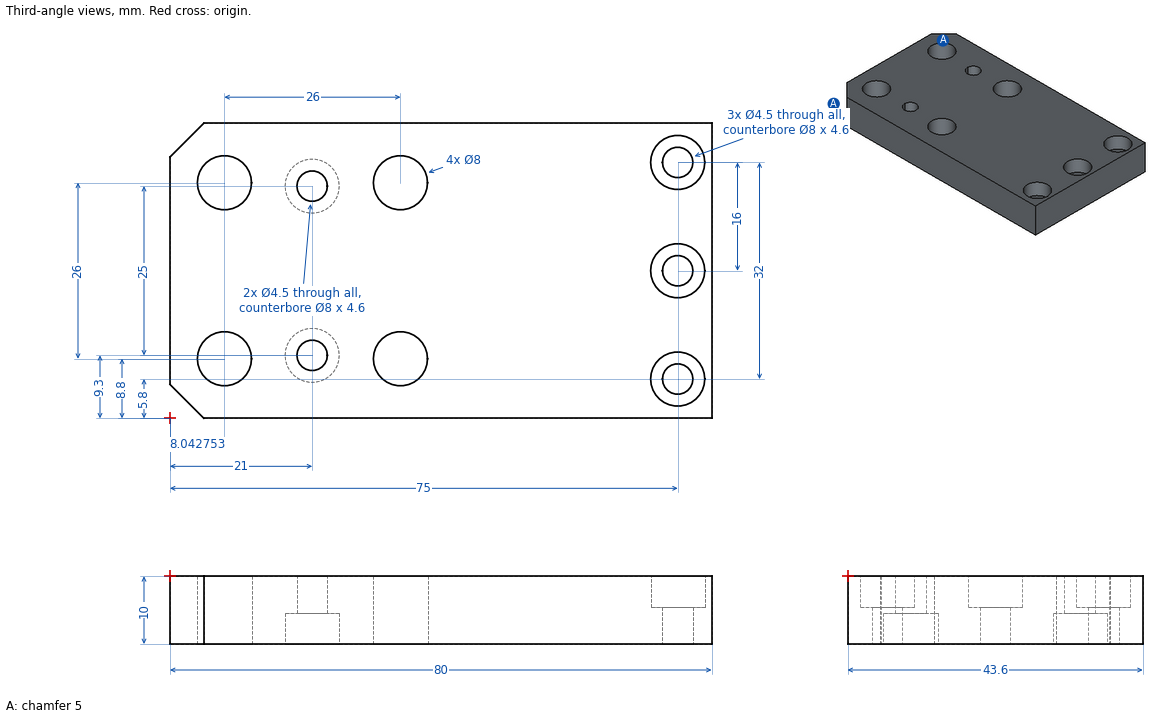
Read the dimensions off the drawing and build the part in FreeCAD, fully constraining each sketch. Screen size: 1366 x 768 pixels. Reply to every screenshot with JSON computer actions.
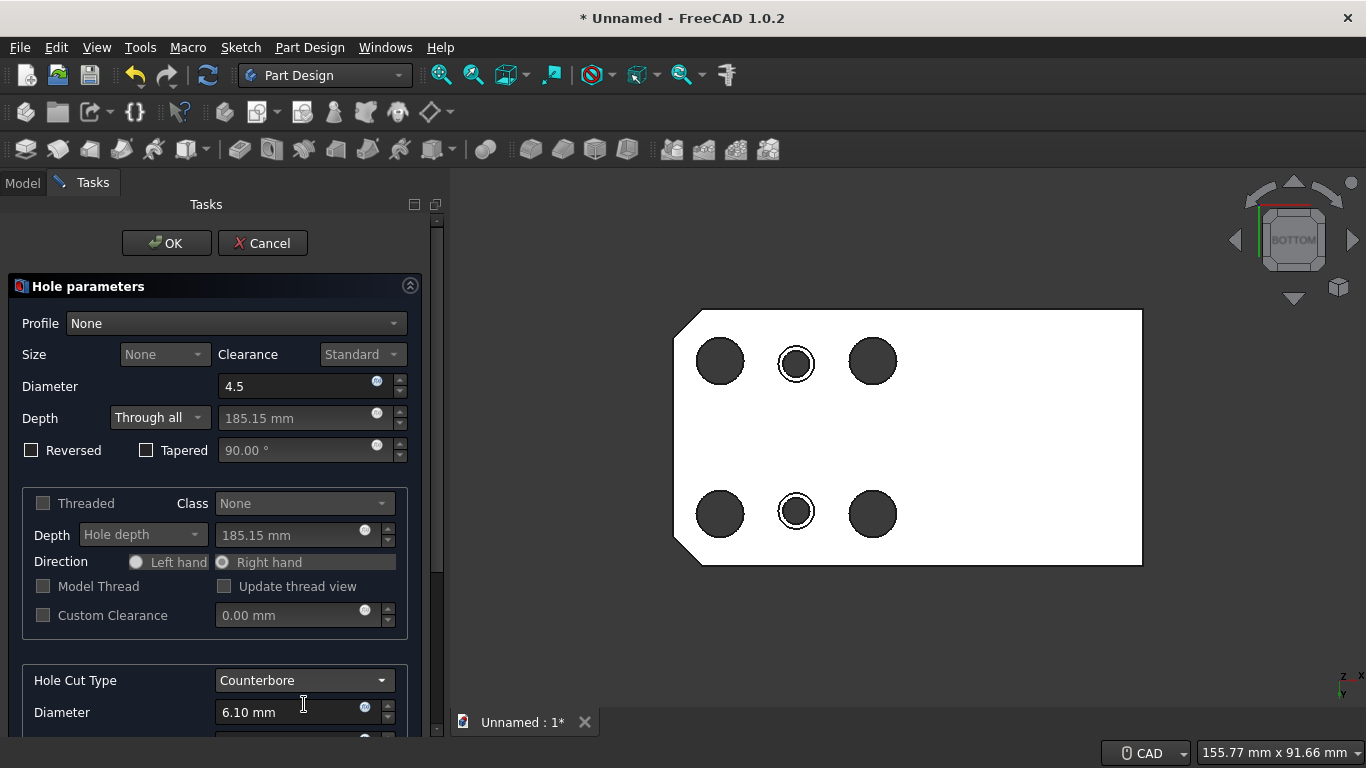
{"action": "triple_click", "coordinate": [298, 712]}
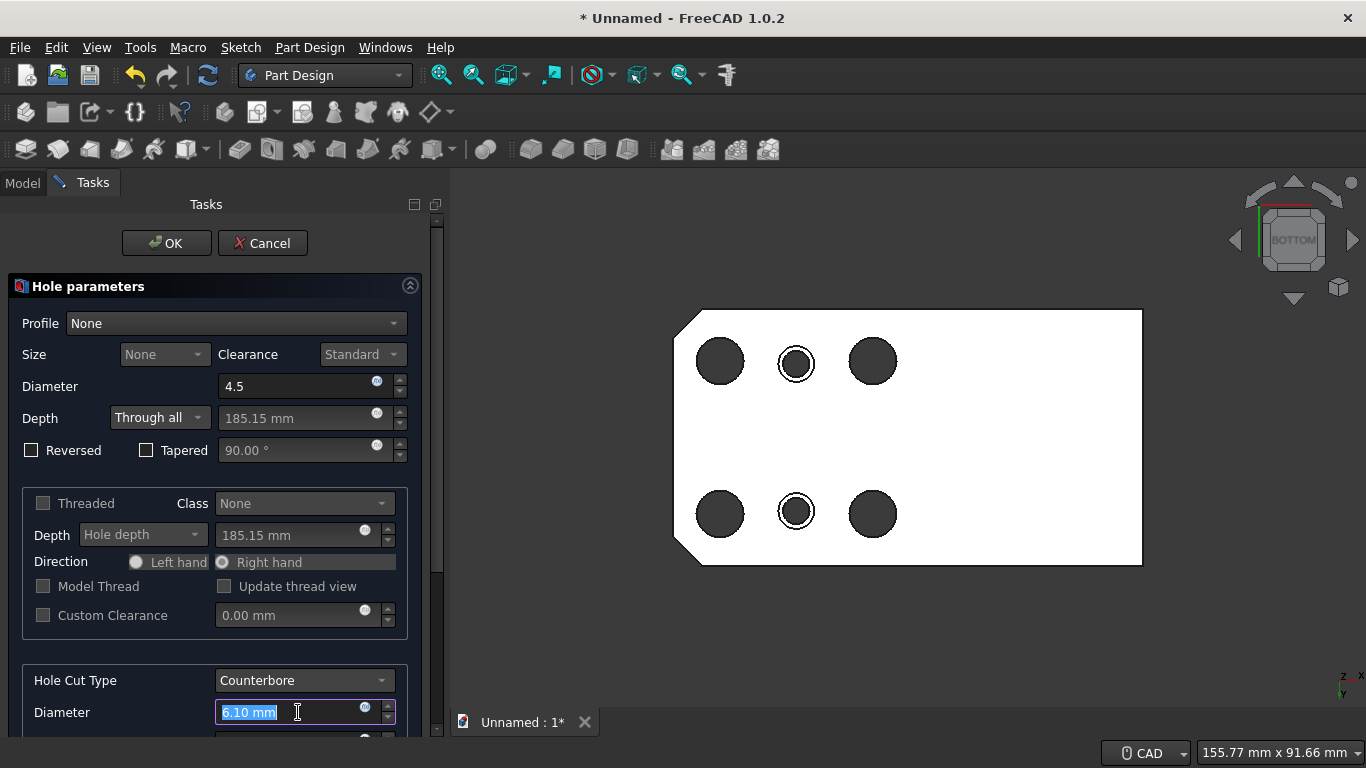
{"action": "type", "text": "8"}
{"action": "key", "text": "Tab"}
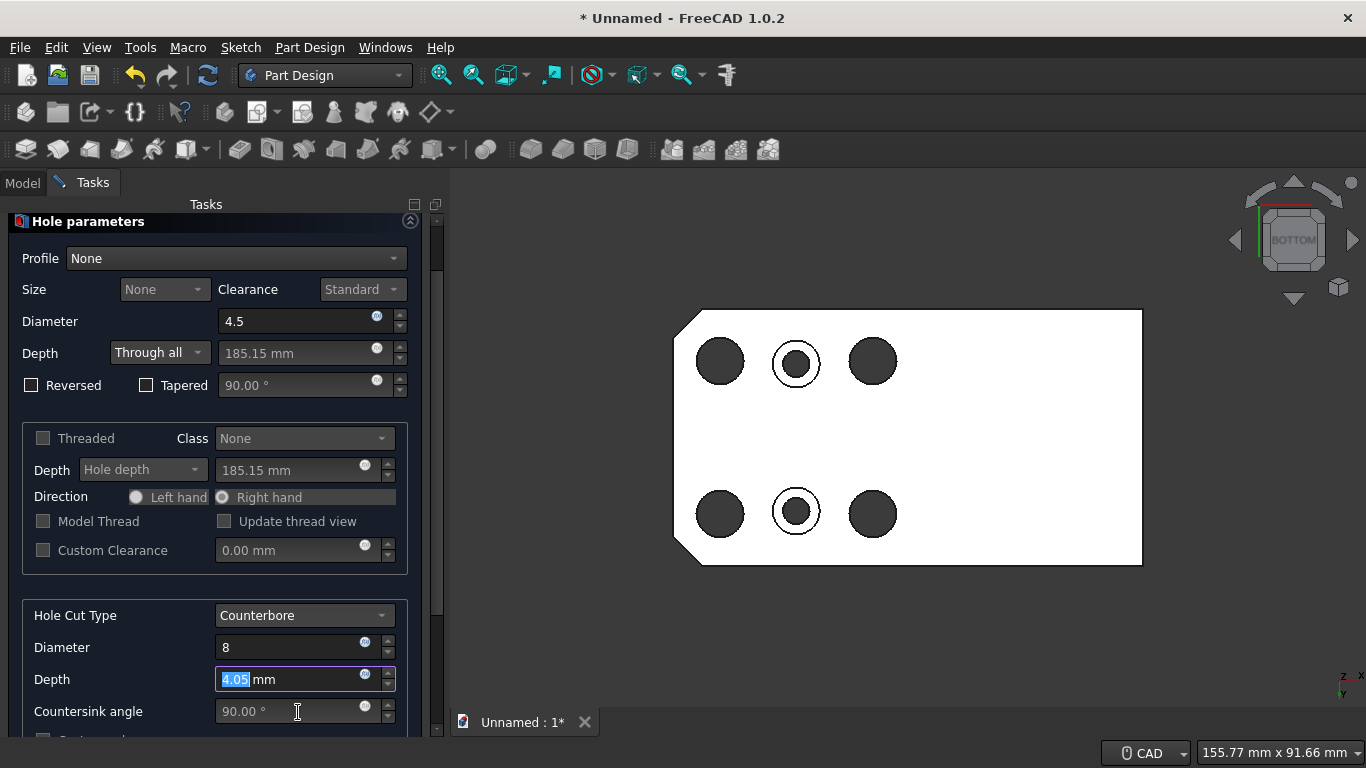
{"action": "type", "text": "4.6"}
{"action": "key", "text": "Tab"}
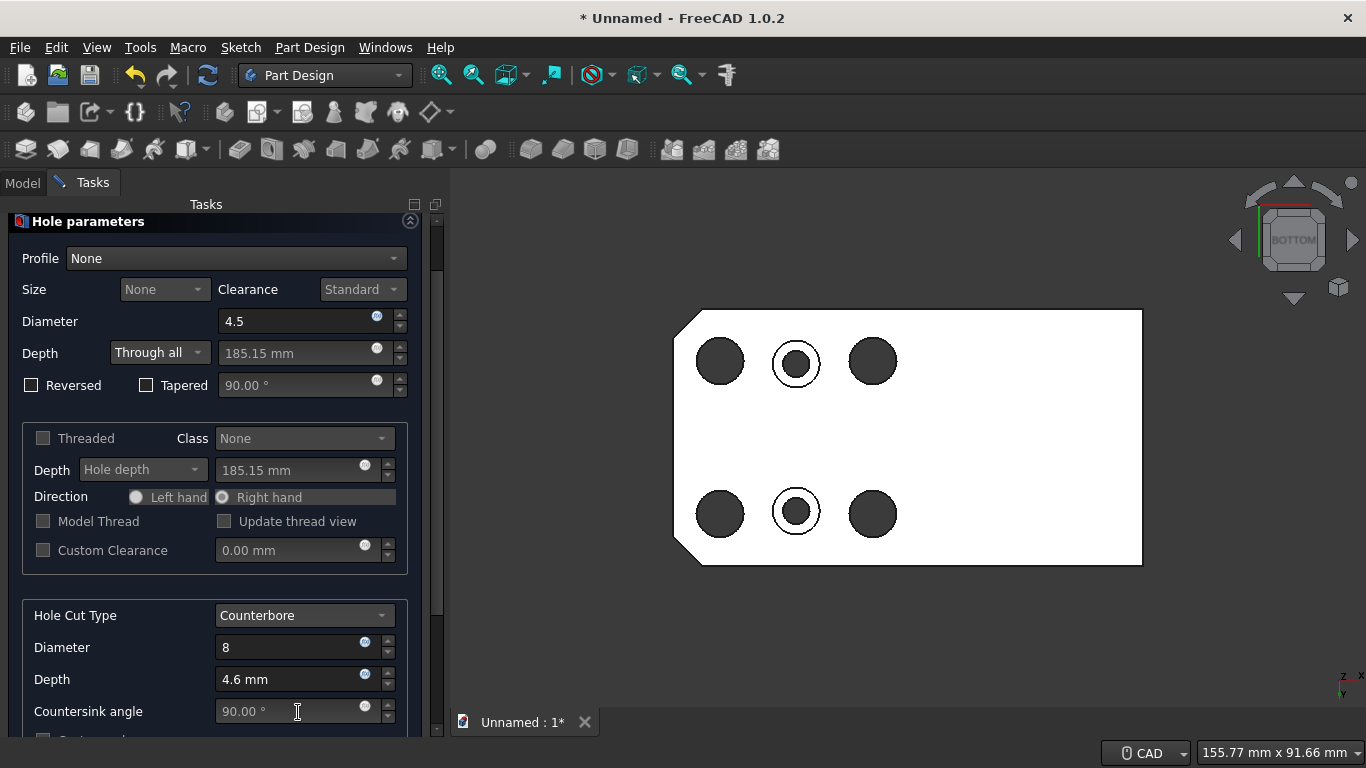
{"action": "scroll", "coordinate": [437, 475], "scroll_direction": "up", "scroll_amount": 2}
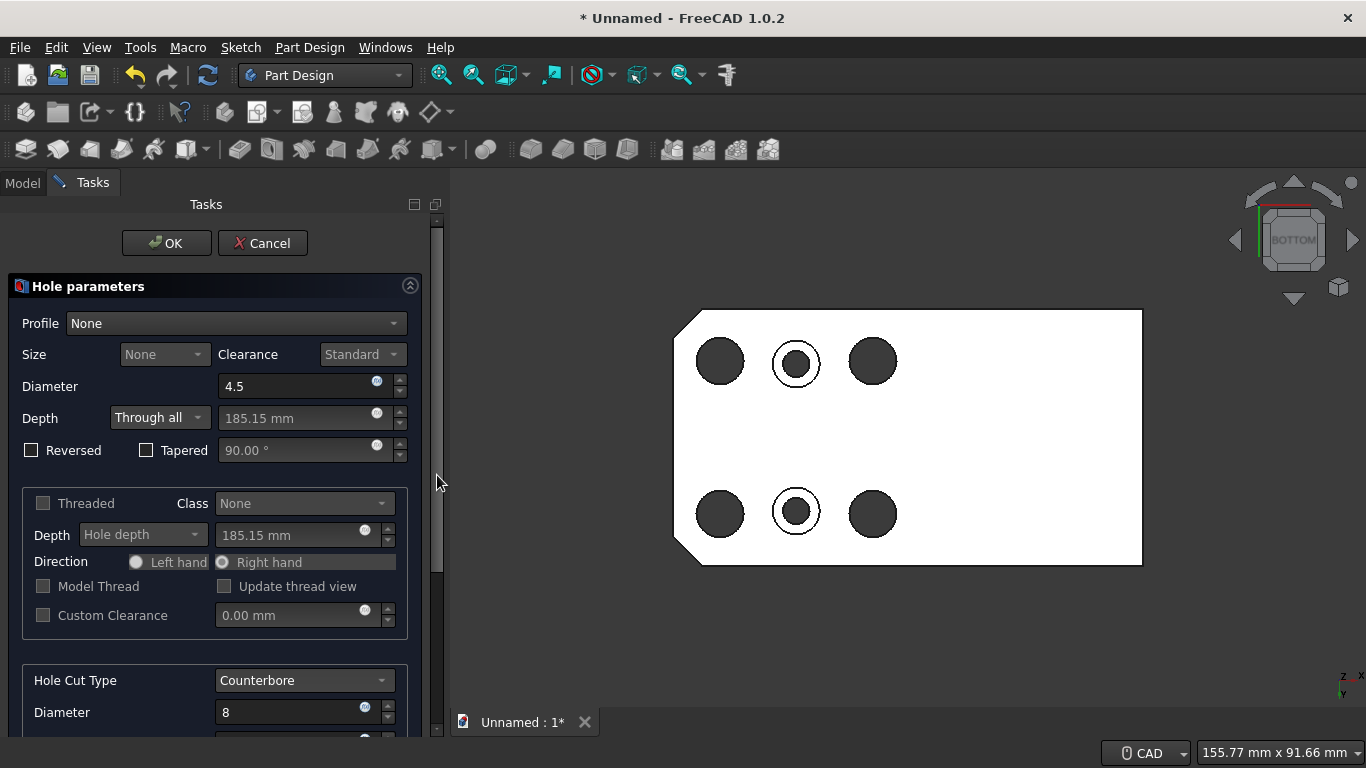
{"action": "left_click", "coordinate": [167, 243]}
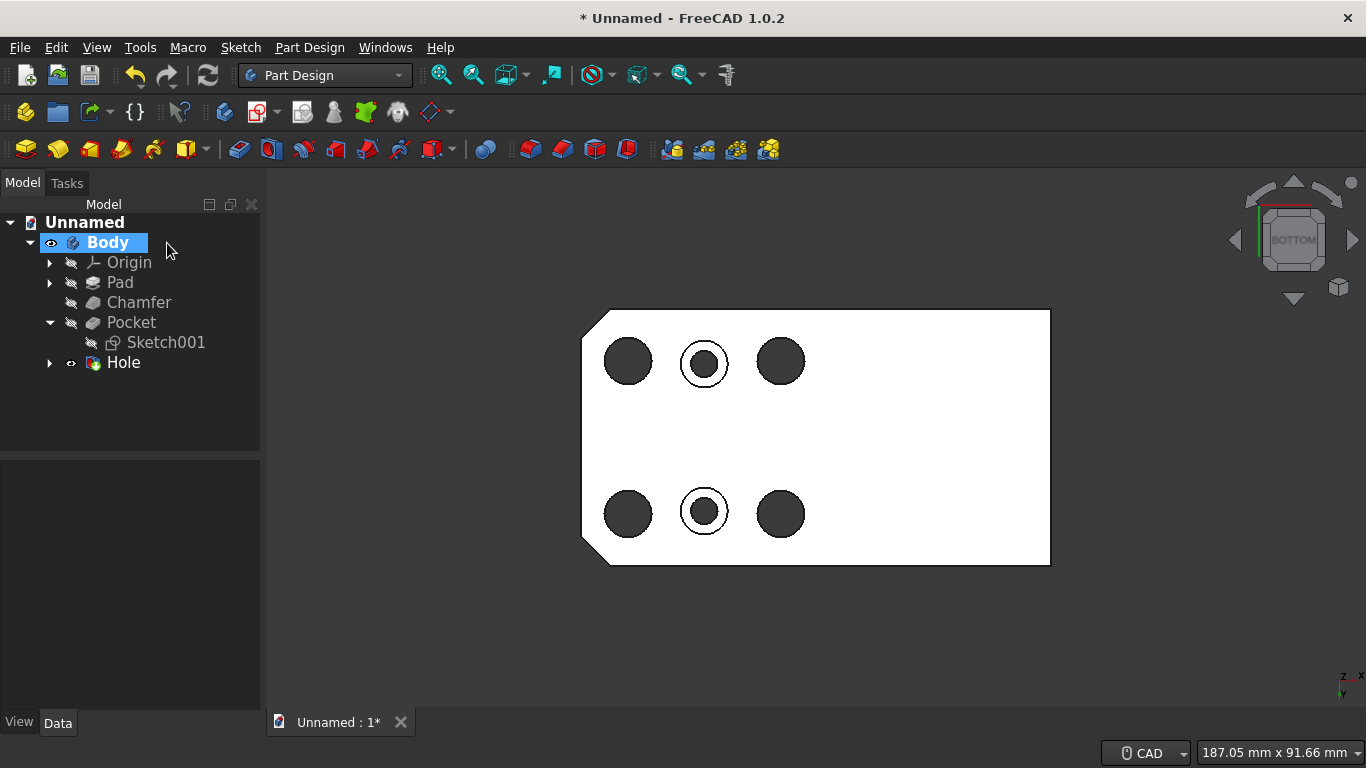
{"action": "key", "text": "0"}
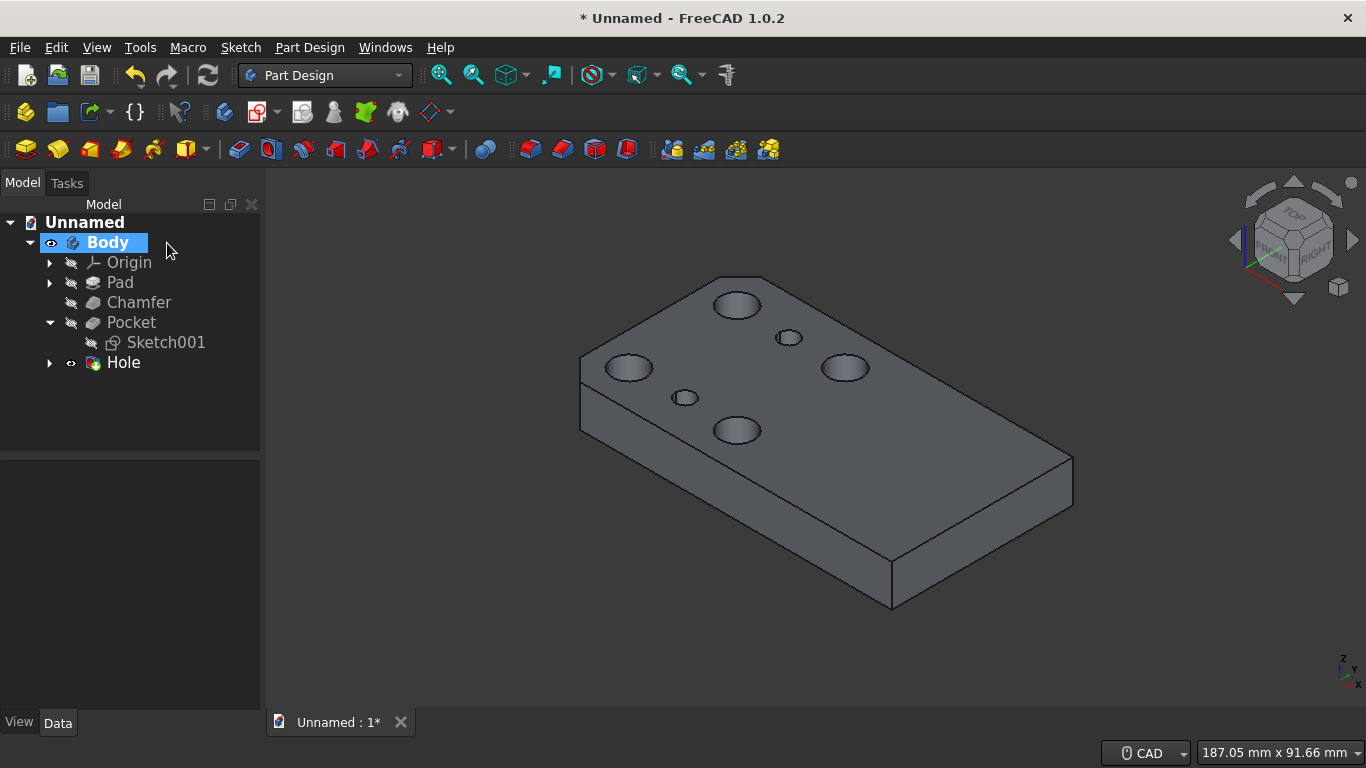
{"action": "left_click", "coordinate": [864, 440]}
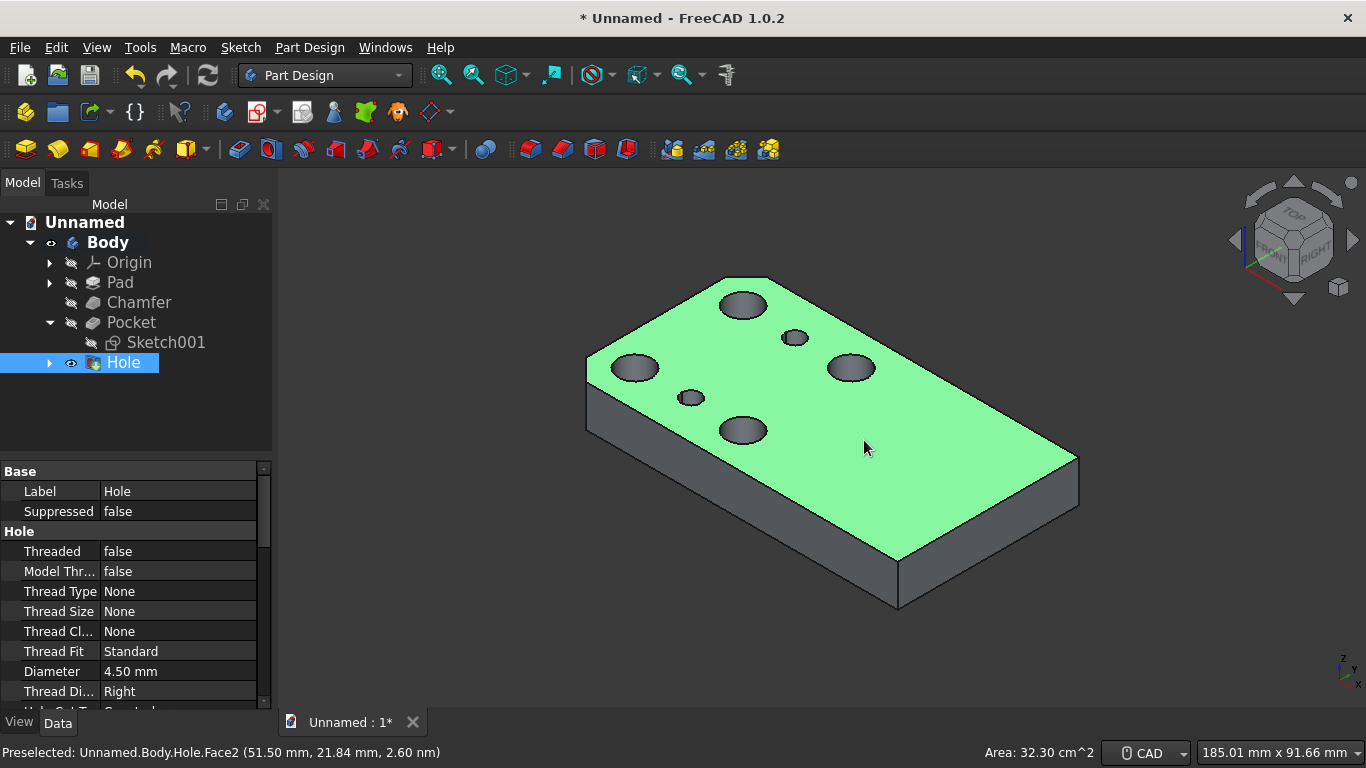
{"action": "left_click", "coordinate": [258, 112]}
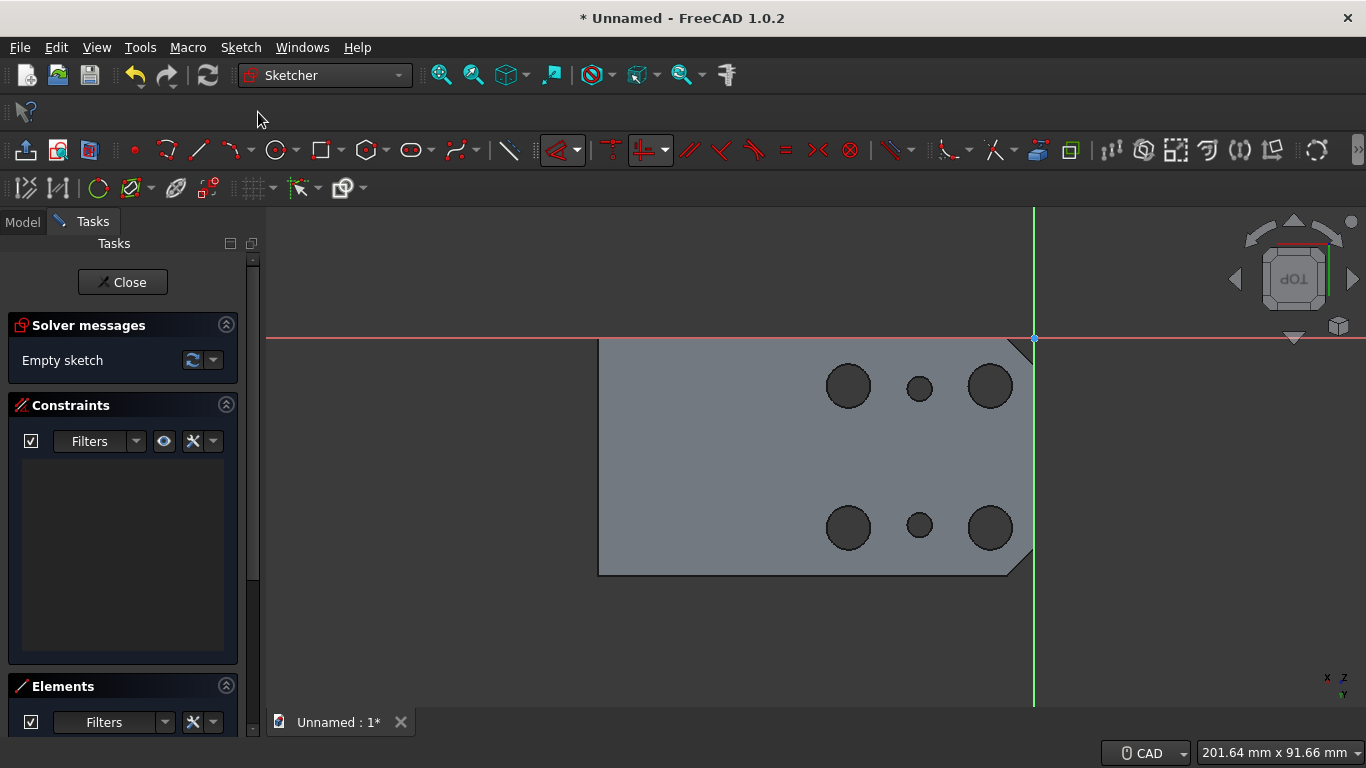
{"action": "scroll", "coordinate": [978, 428], "scroll_direction": "up", "scroll_amount": 2}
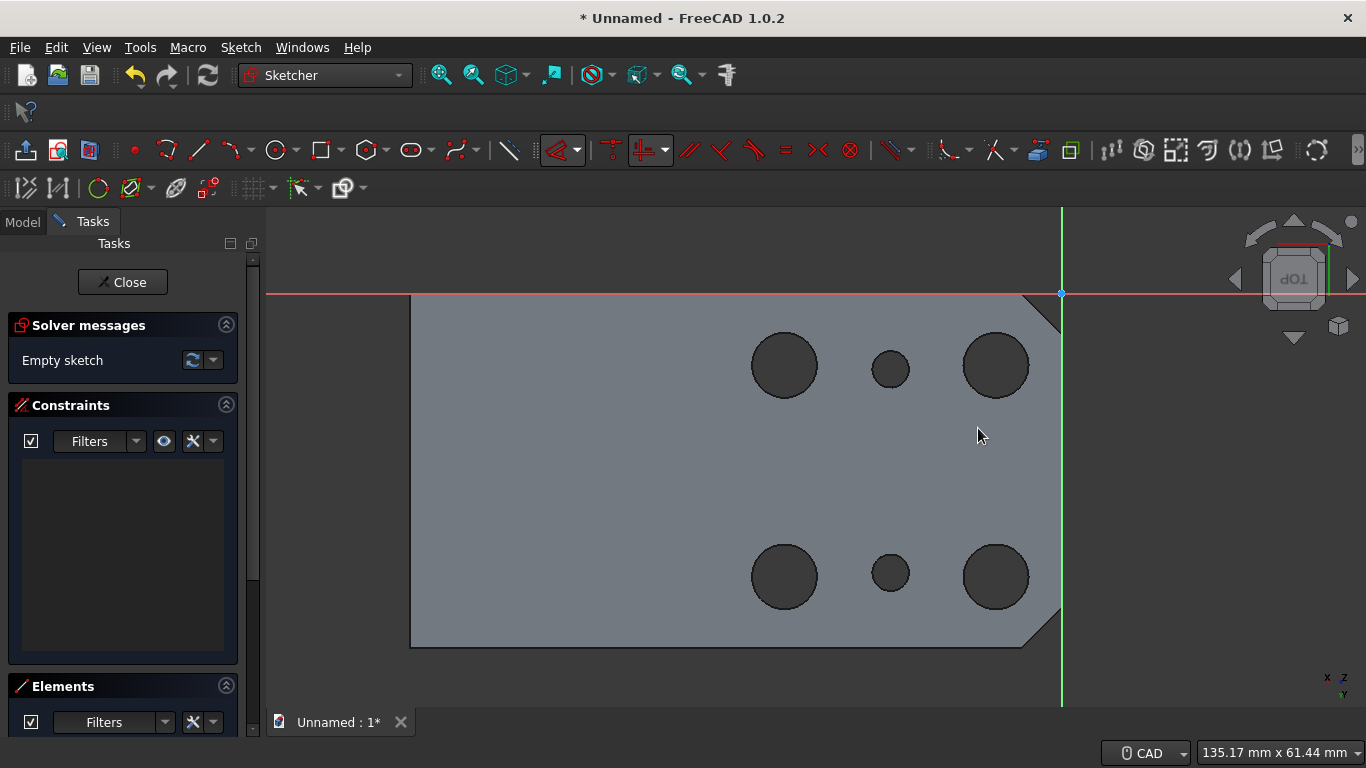
{"action": "left_click", "coordinate": [276, 150]}